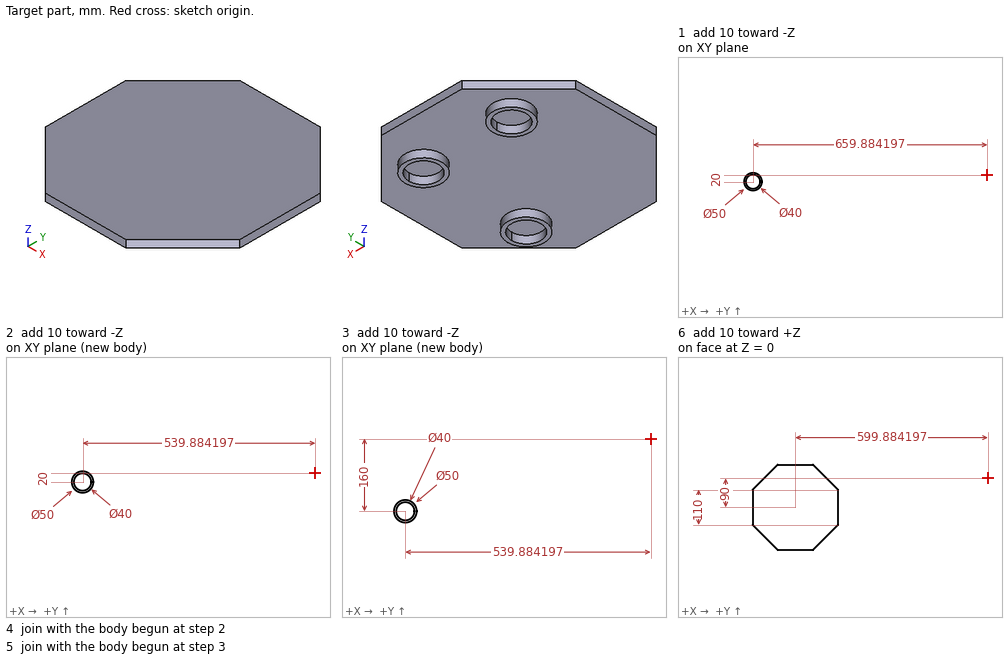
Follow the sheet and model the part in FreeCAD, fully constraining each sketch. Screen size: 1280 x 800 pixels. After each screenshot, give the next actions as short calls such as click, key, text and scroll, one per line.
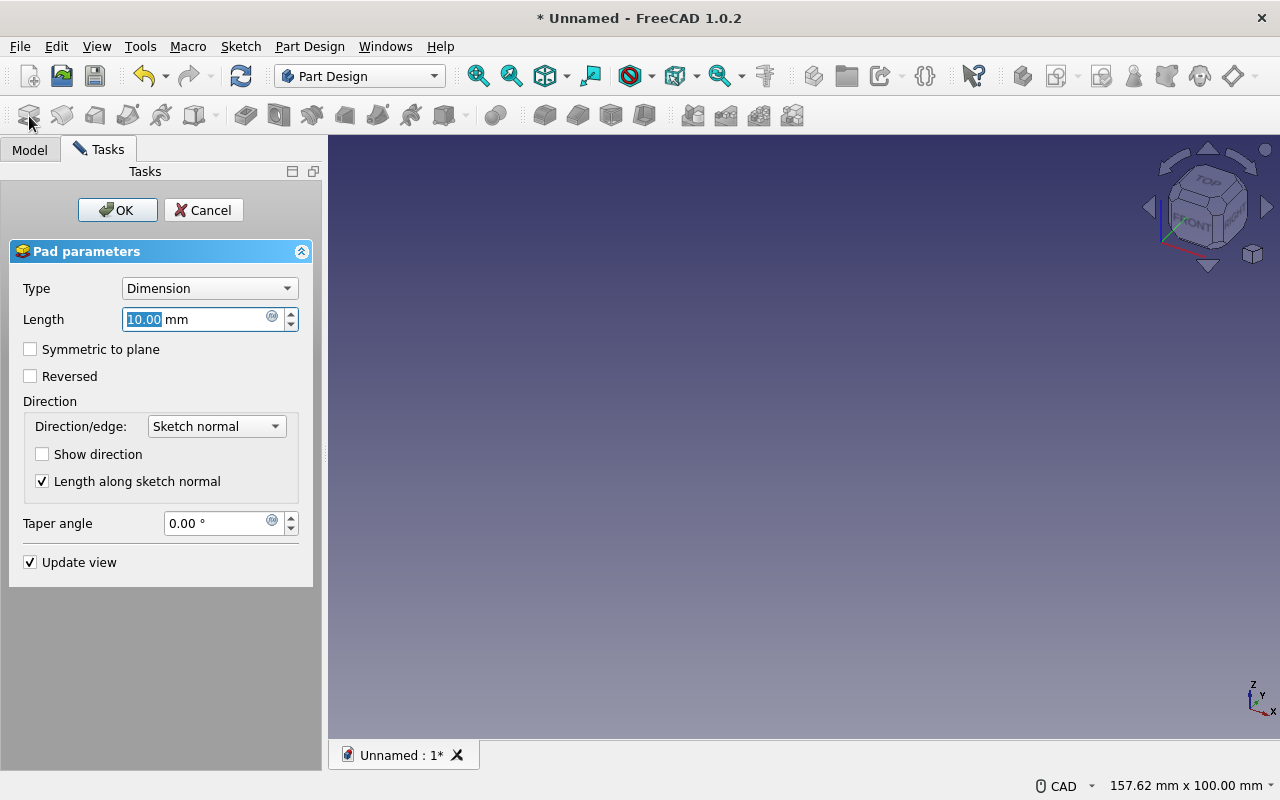
text(10)
key(Tab)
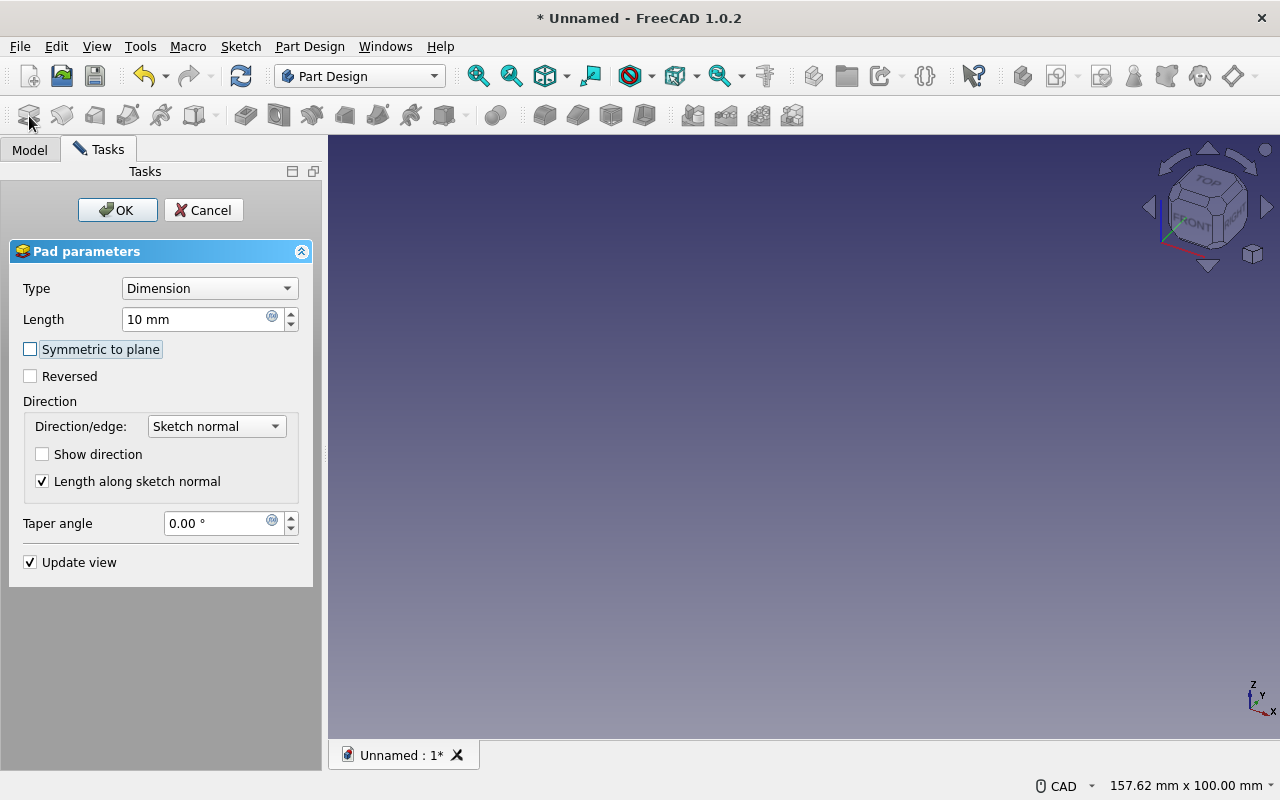
click(31, 376)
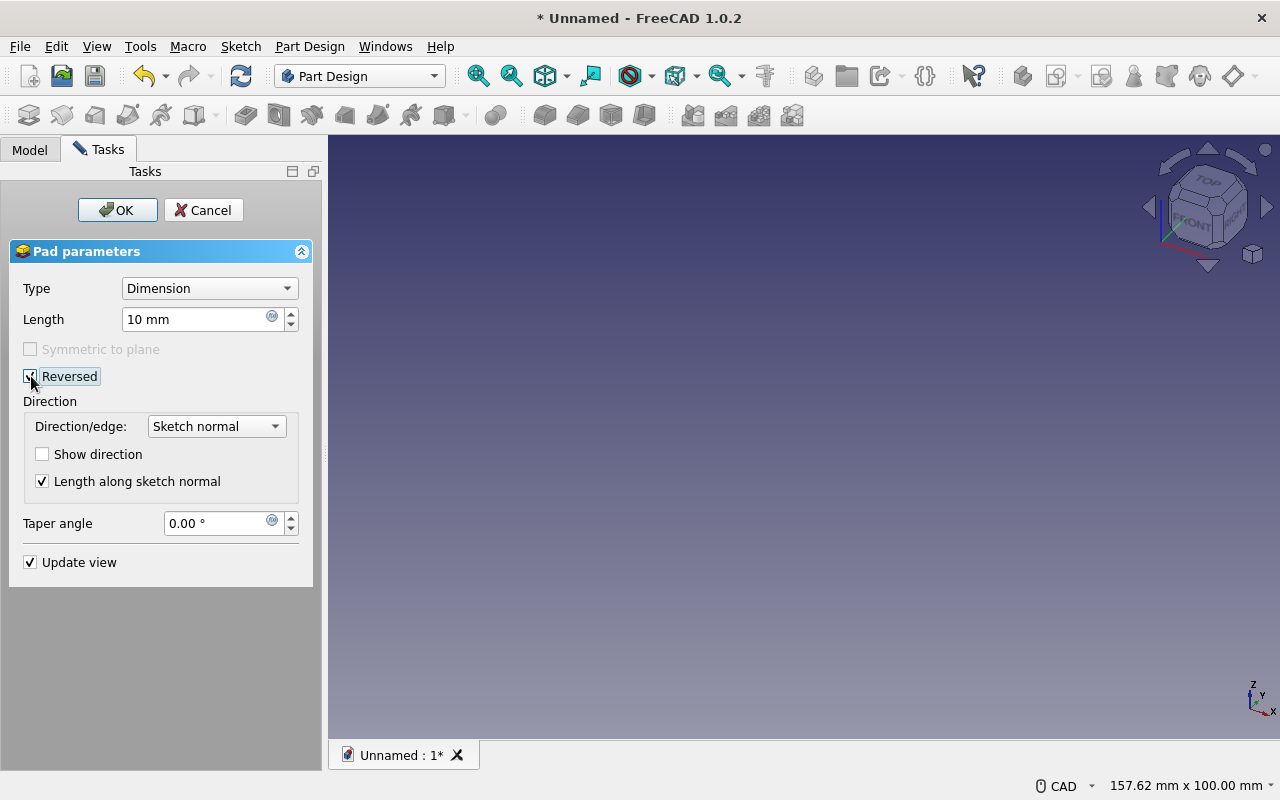
click(118, 210)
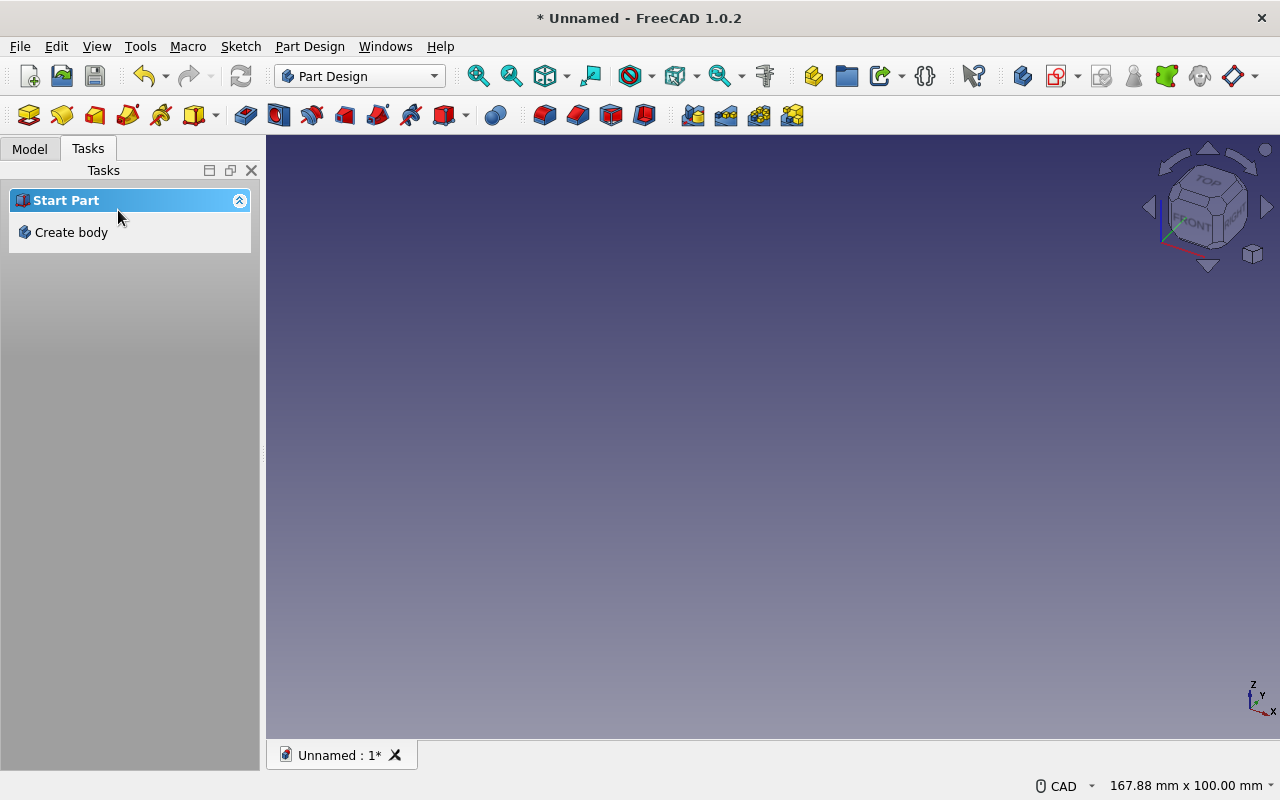
key(v)
key(f)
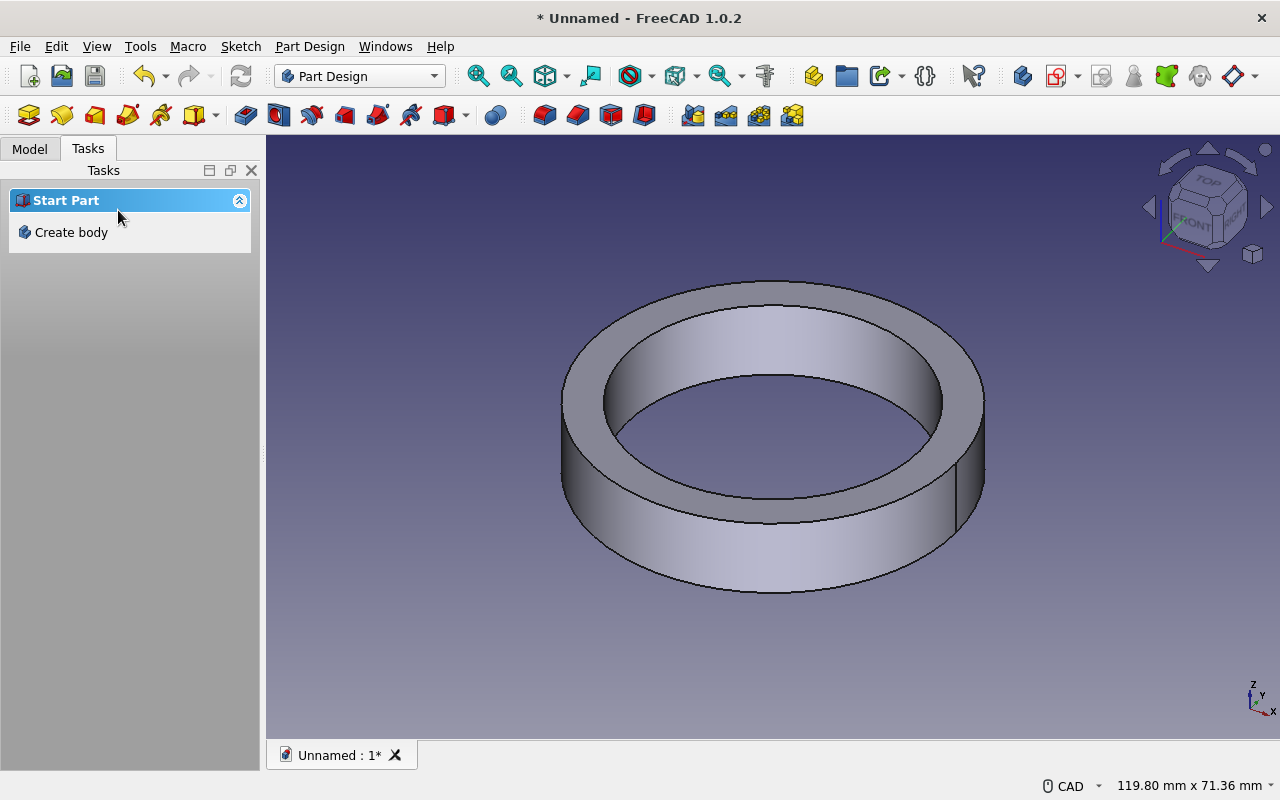
click(1023, 76)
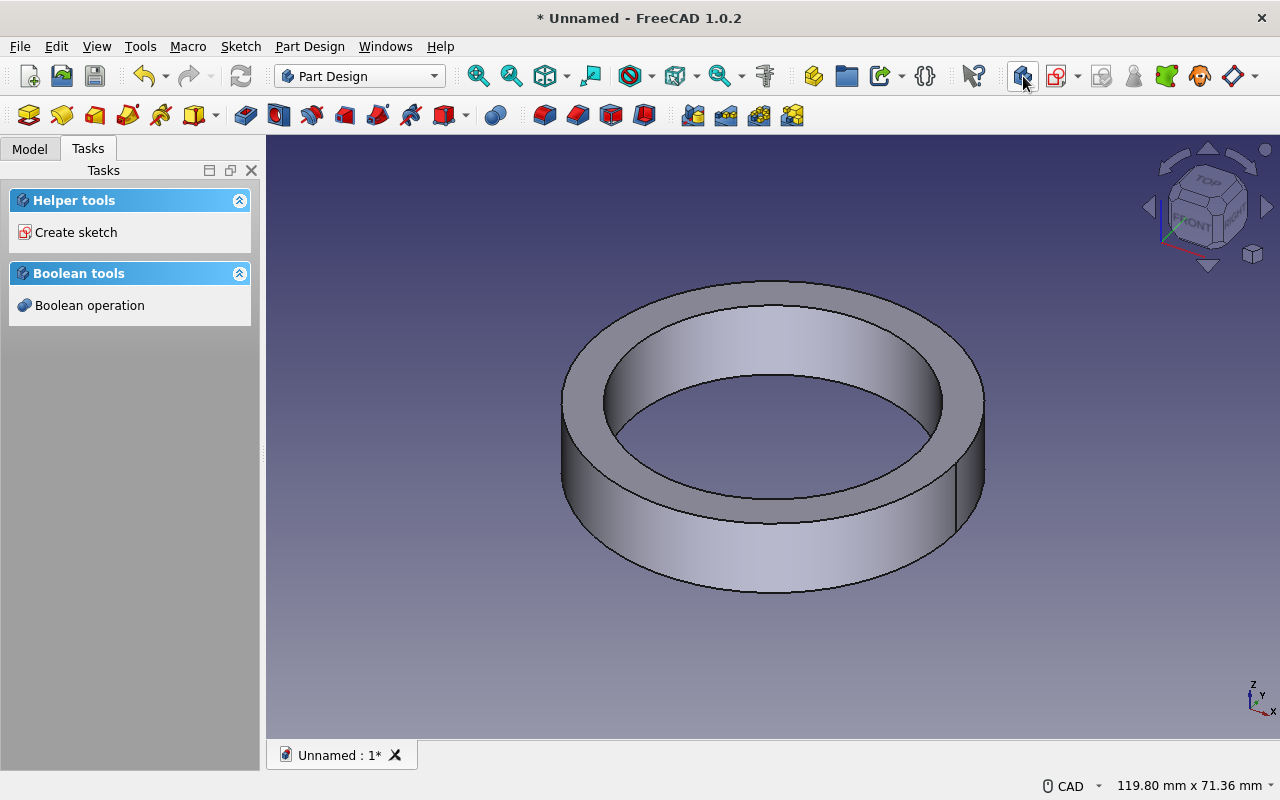
click(306, 699)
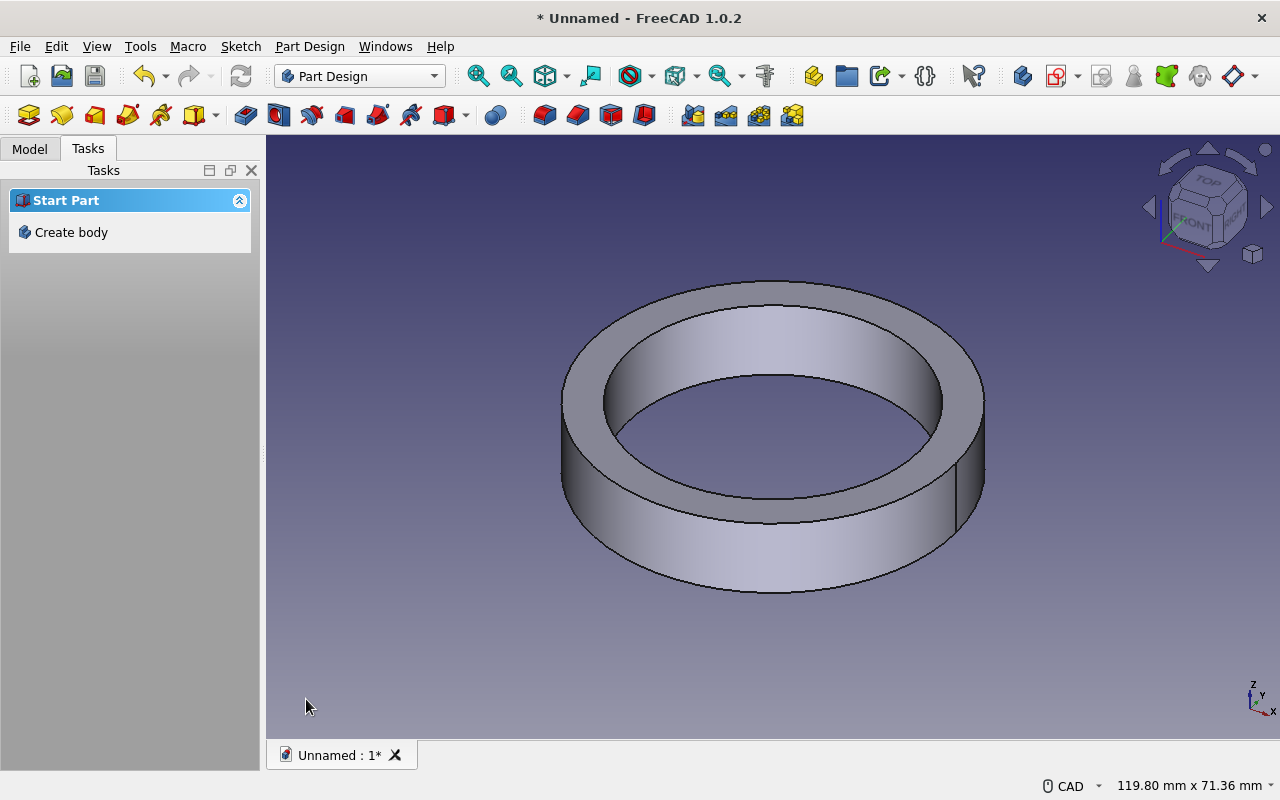
click(1056, 76)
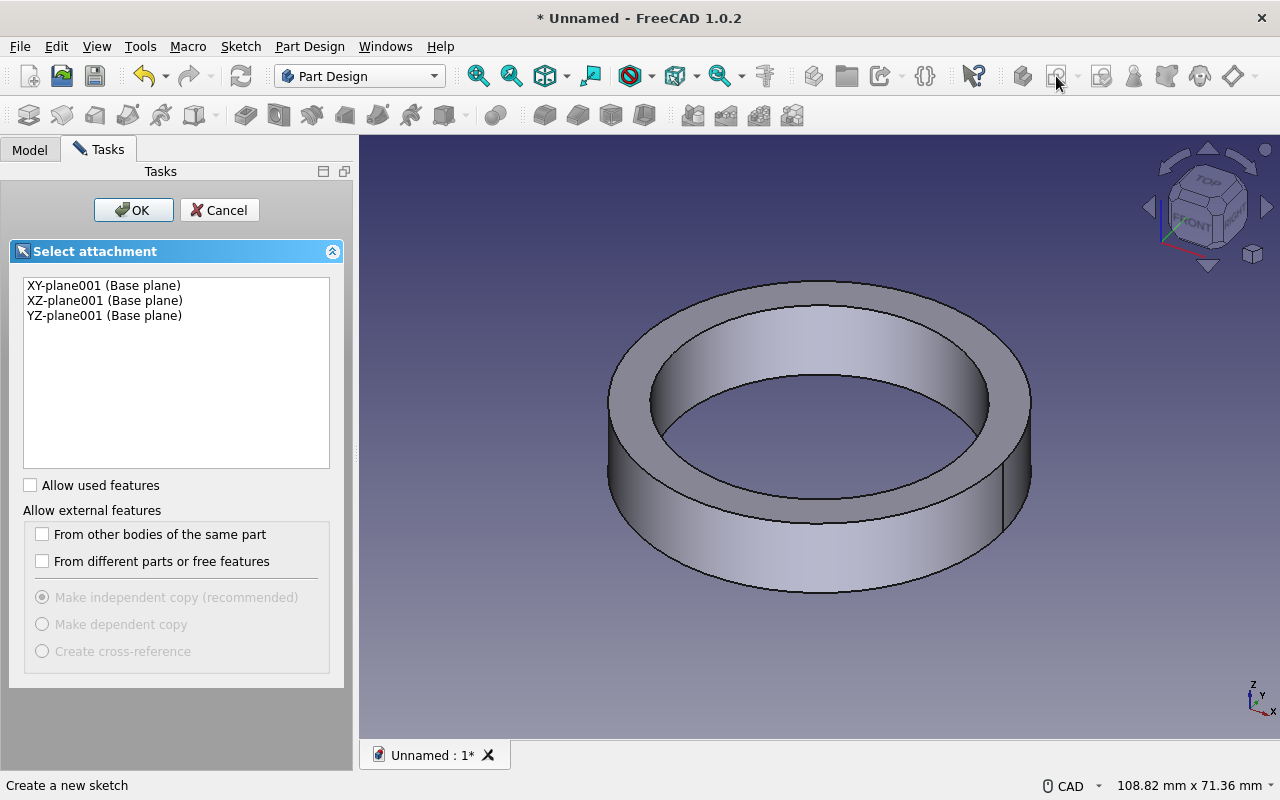
click(84, 286)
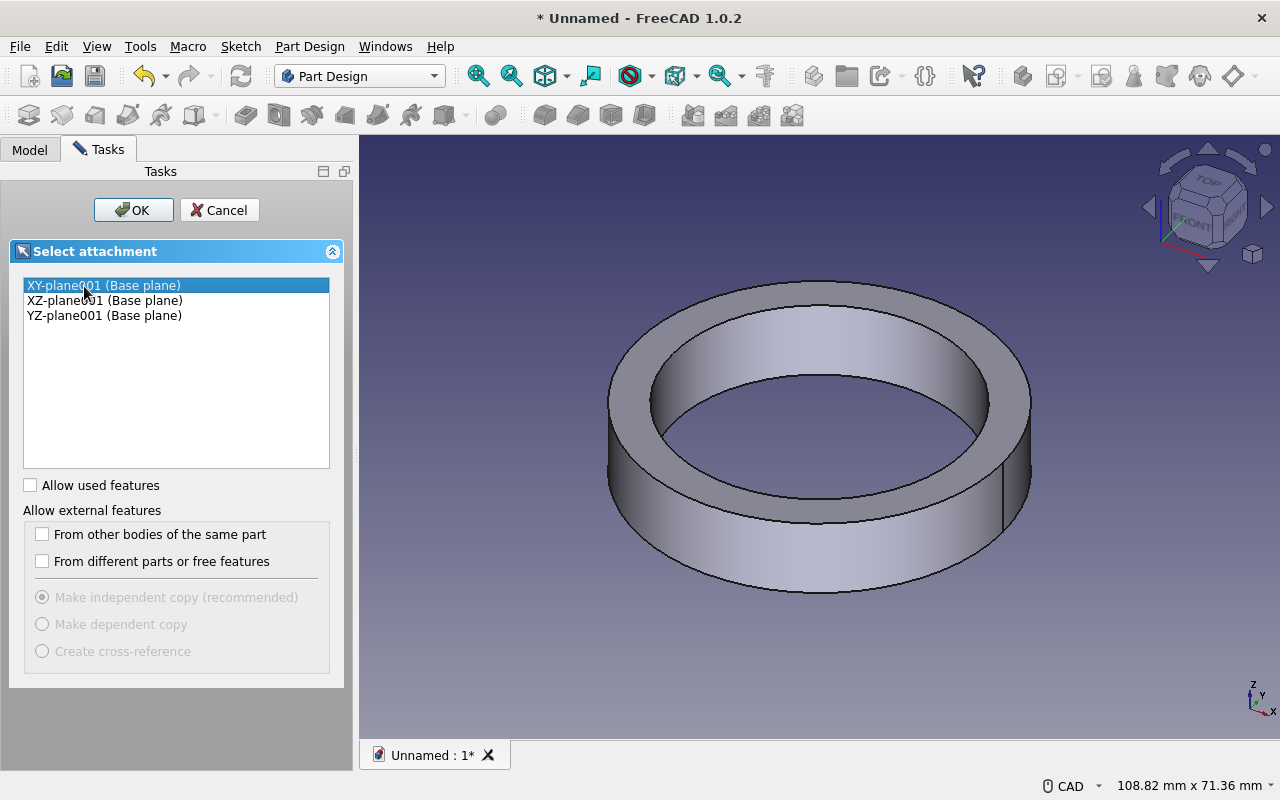
click(134, 210)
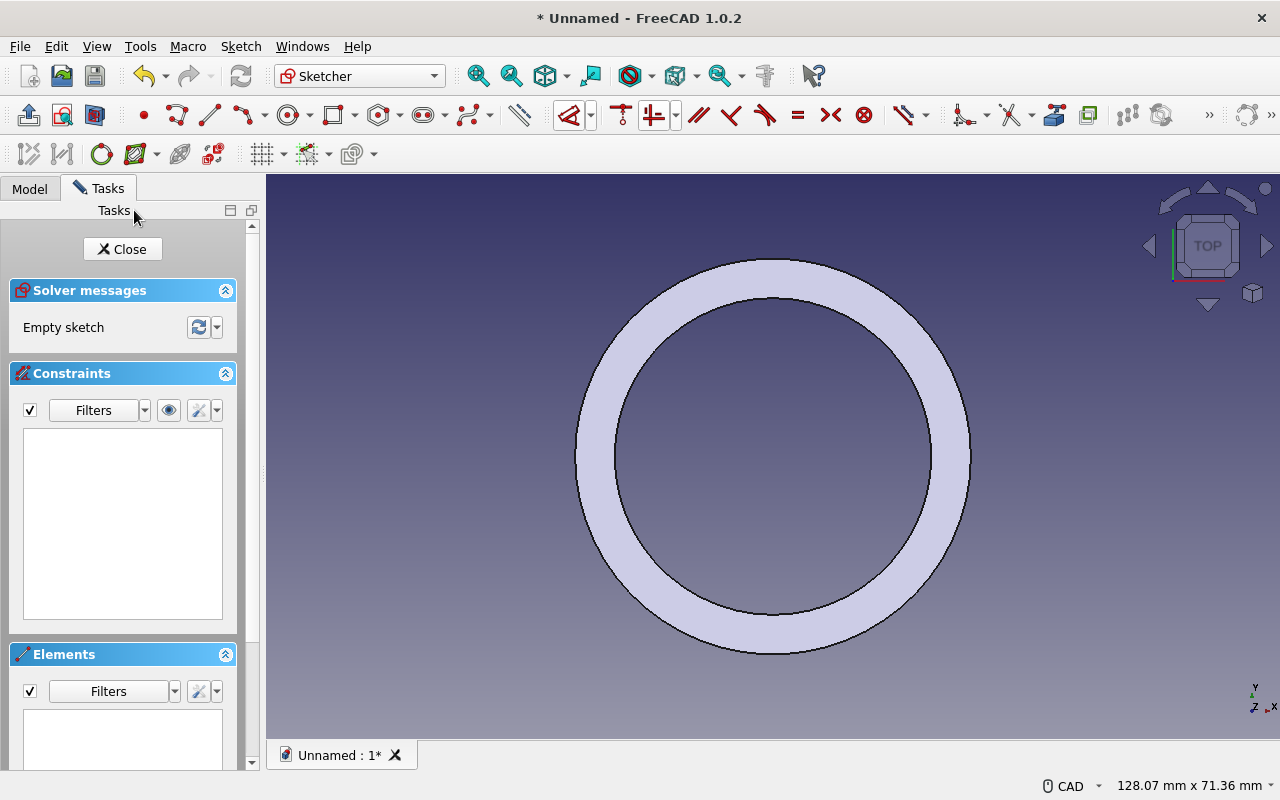
scroll(704, 456, down, 5)